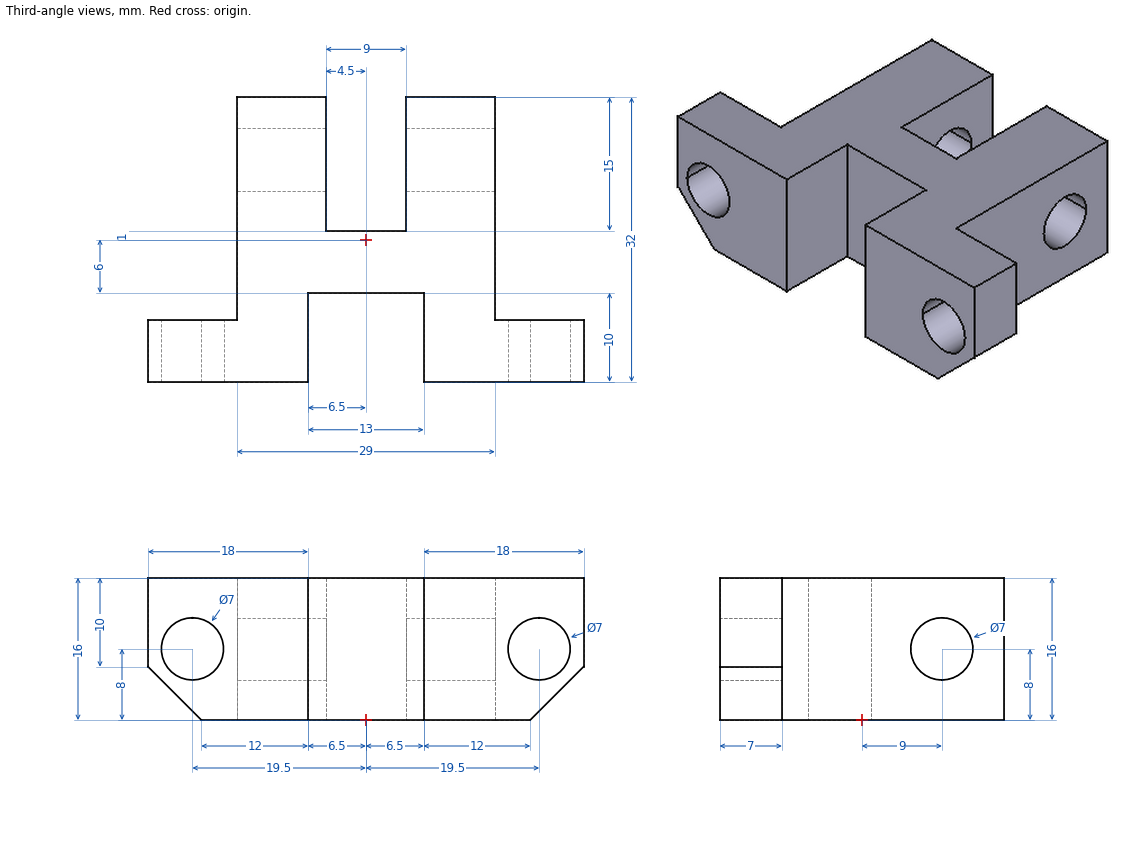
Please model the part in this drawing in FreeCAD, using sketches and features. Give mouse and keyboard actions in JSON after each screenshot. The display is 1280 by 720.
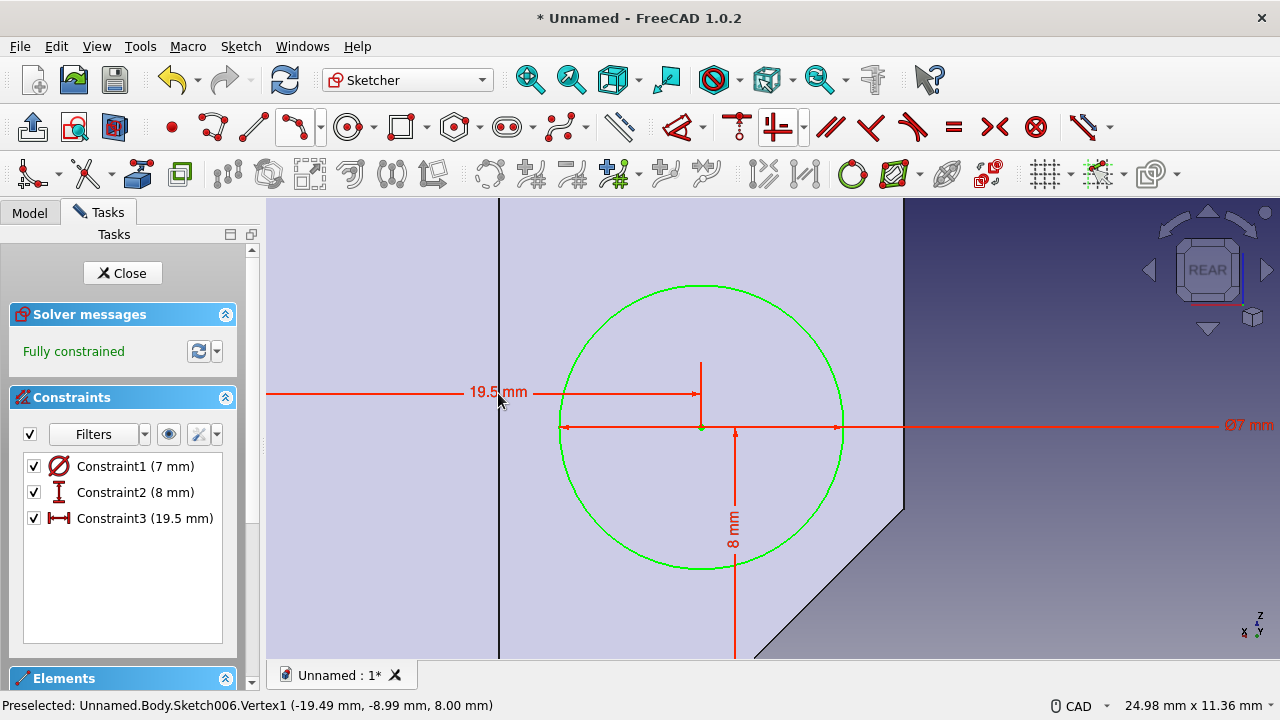
{"action": "left_click", "coordinate": [123, 273]}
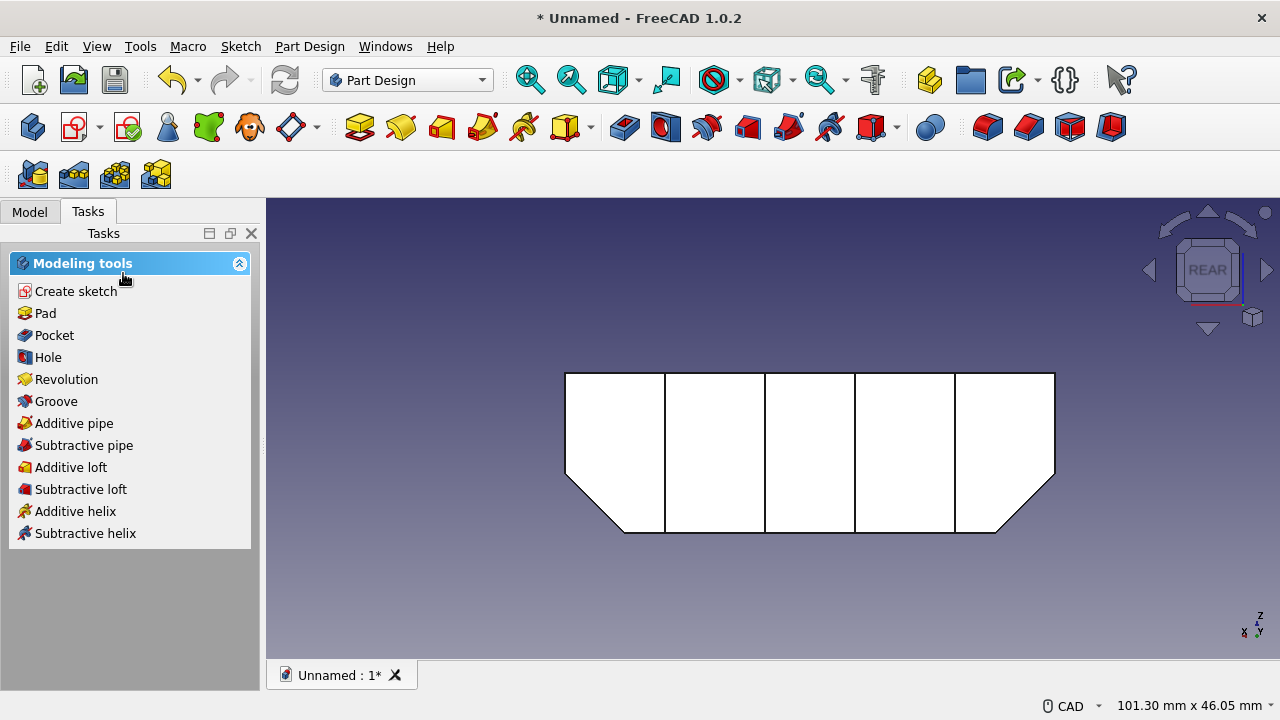
{"action": "left_click", "coordinate": [625, 128]}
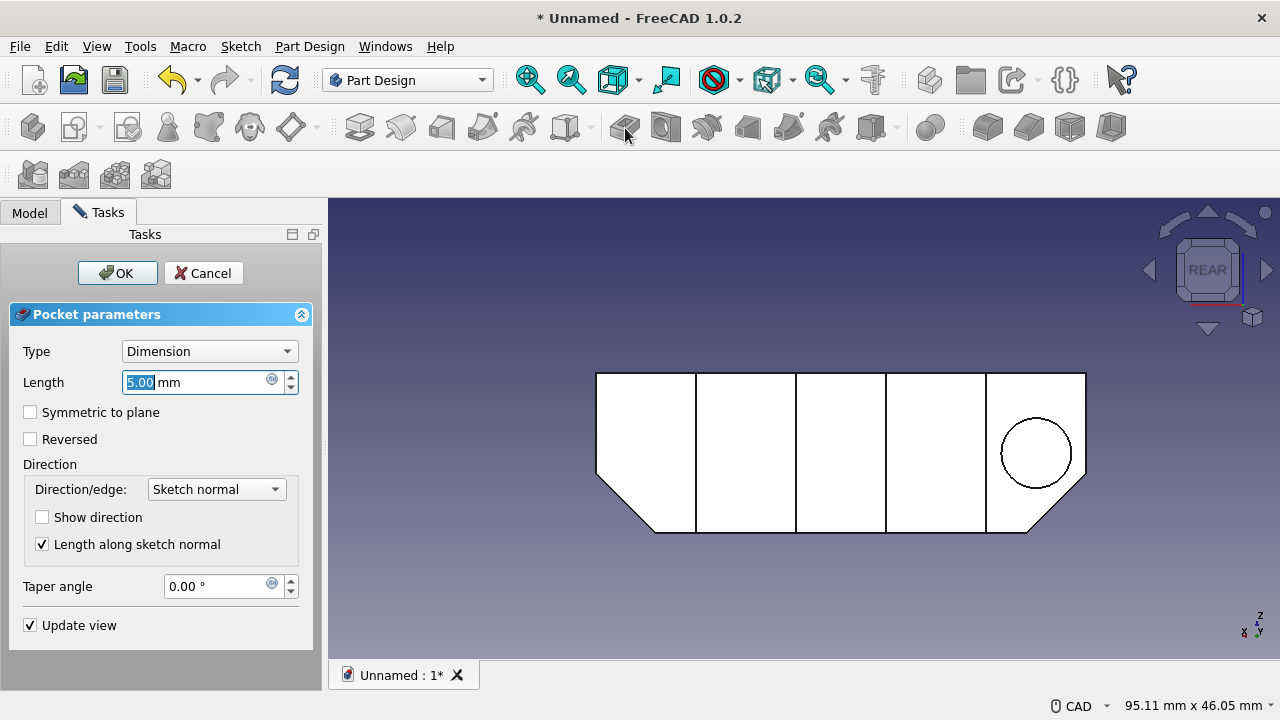
{"action": "type", "text": "7"}
{"action": "key", "text": "Tab"}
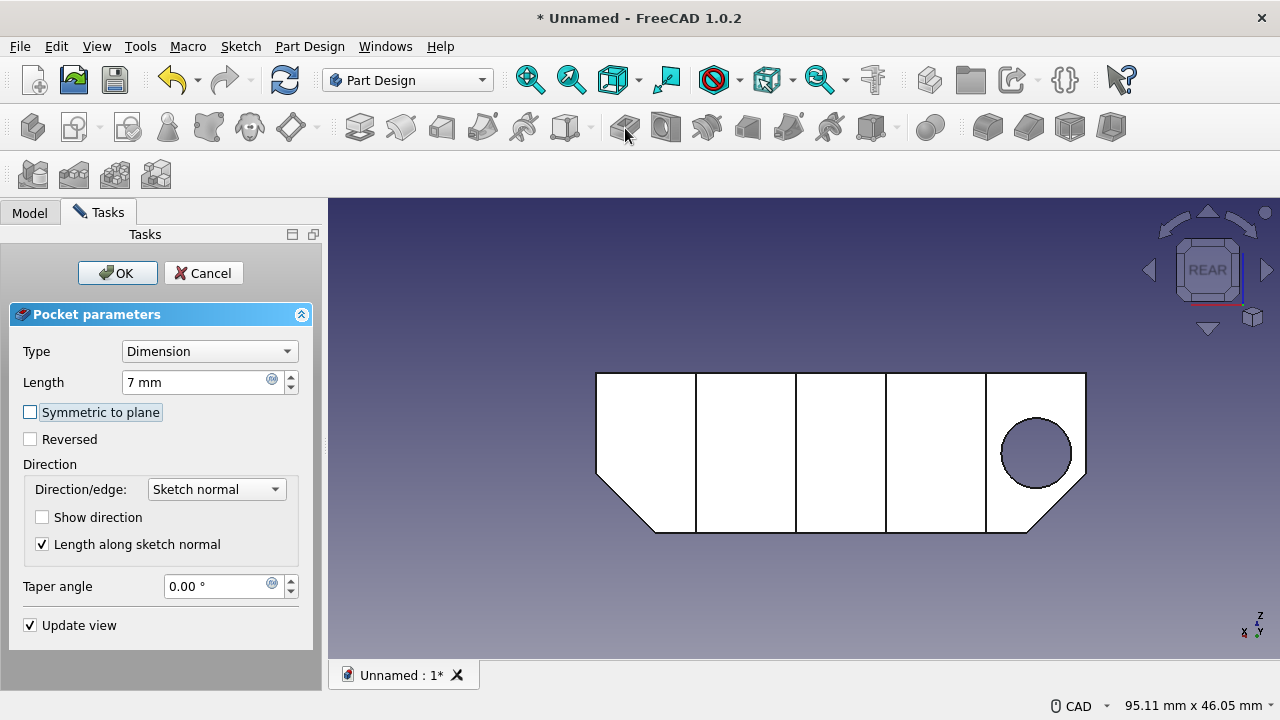
{"action": "left_click", "coordinate": [118, 273]}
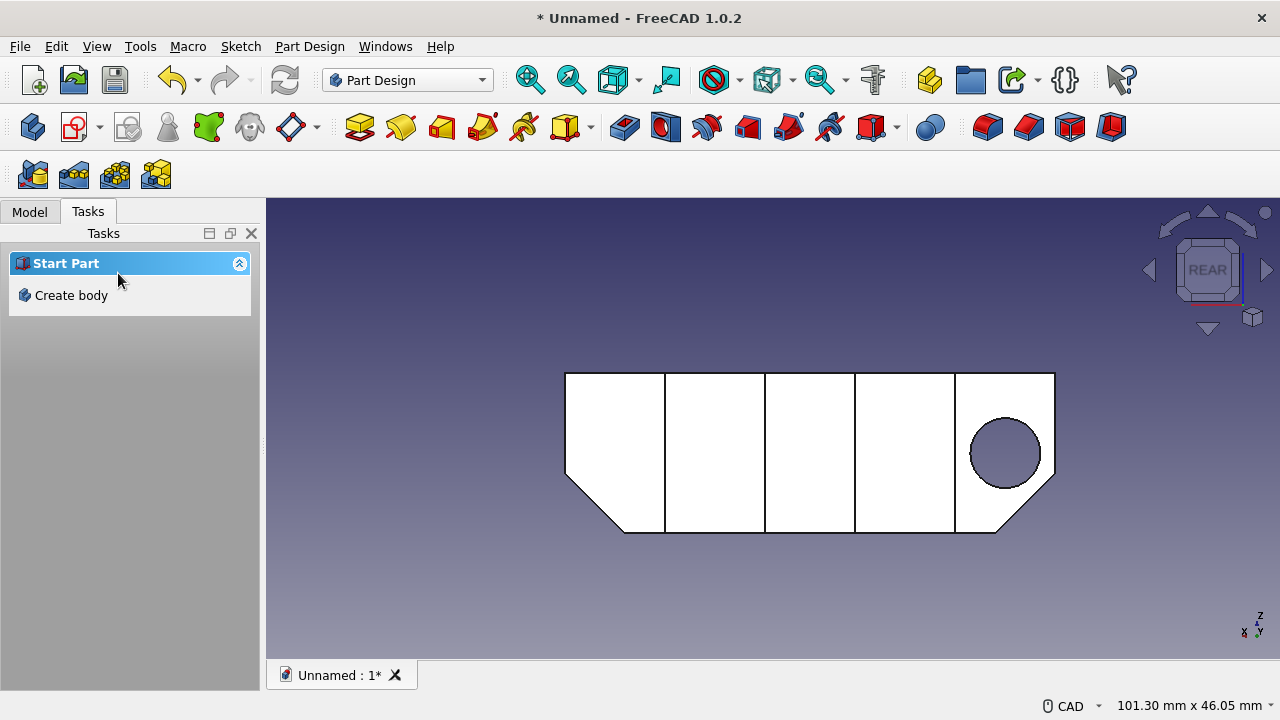
{"action": "left_click", "coordinate": [615, 429]}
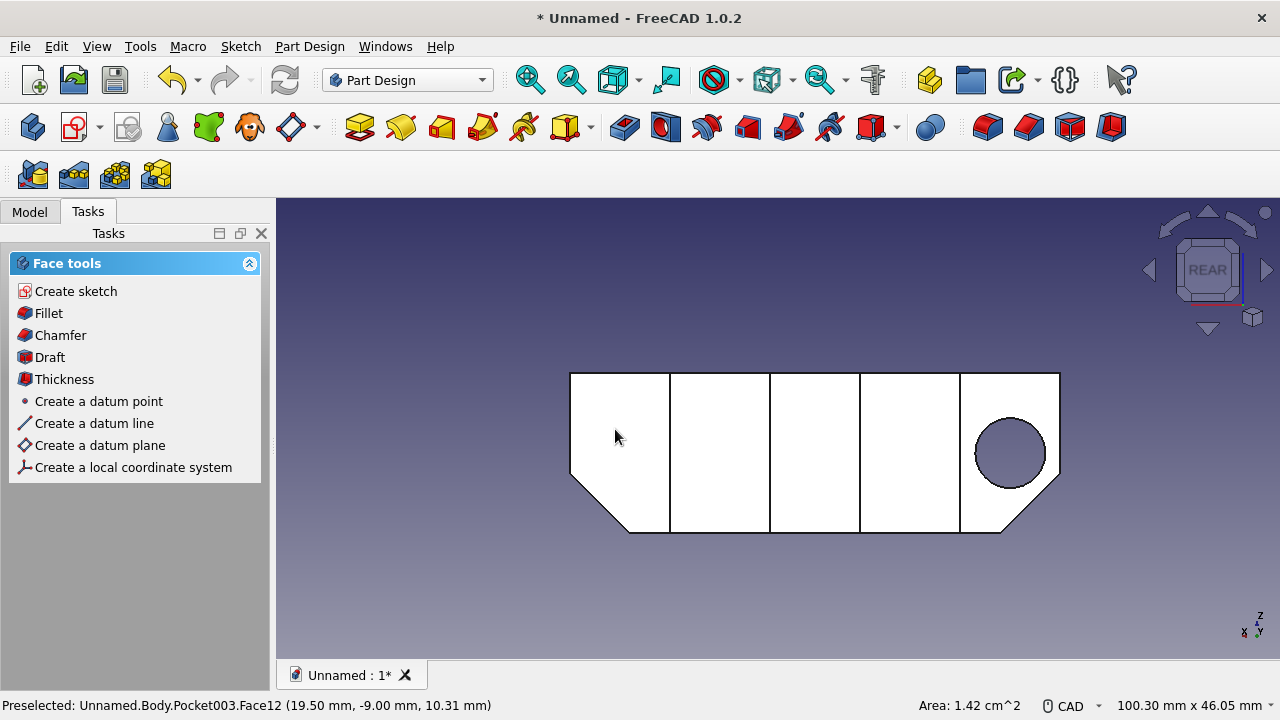
{"action": "left_click", "coordinate": [74, 128]}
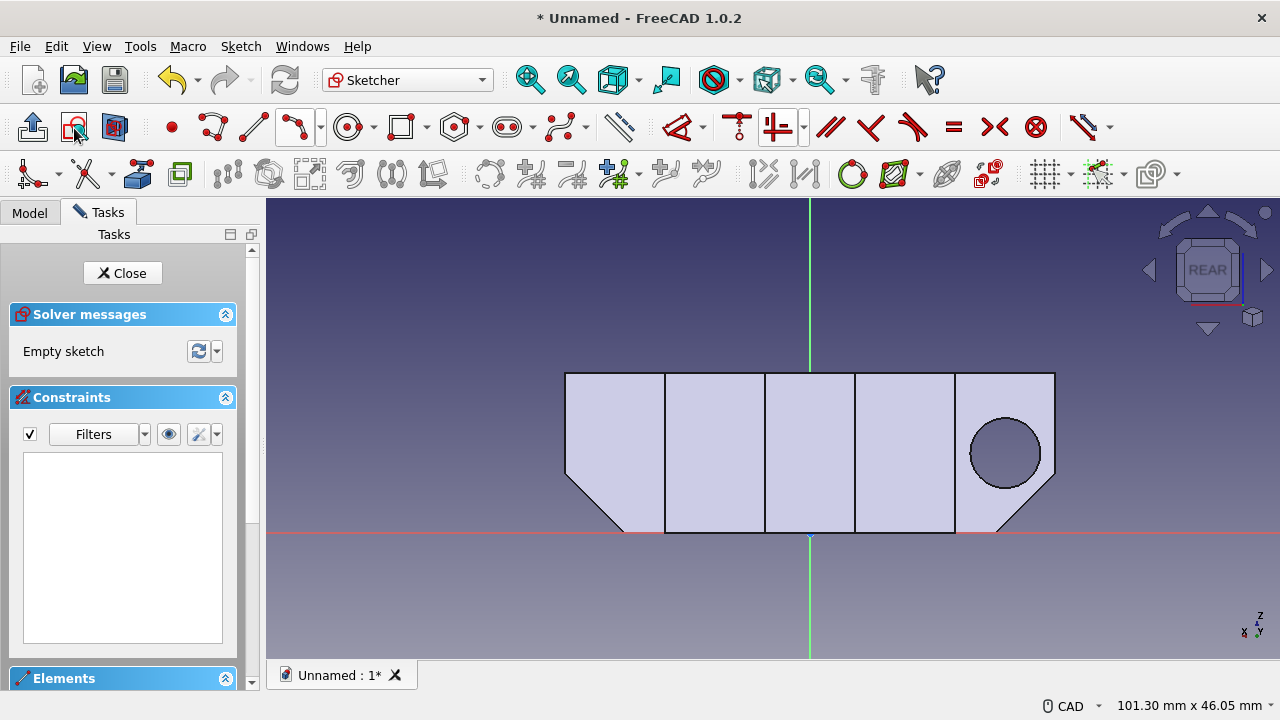
{"action": "scroll", "coordinate": [586, 461], "scroll_direction": "up", "scroll_amount": 7}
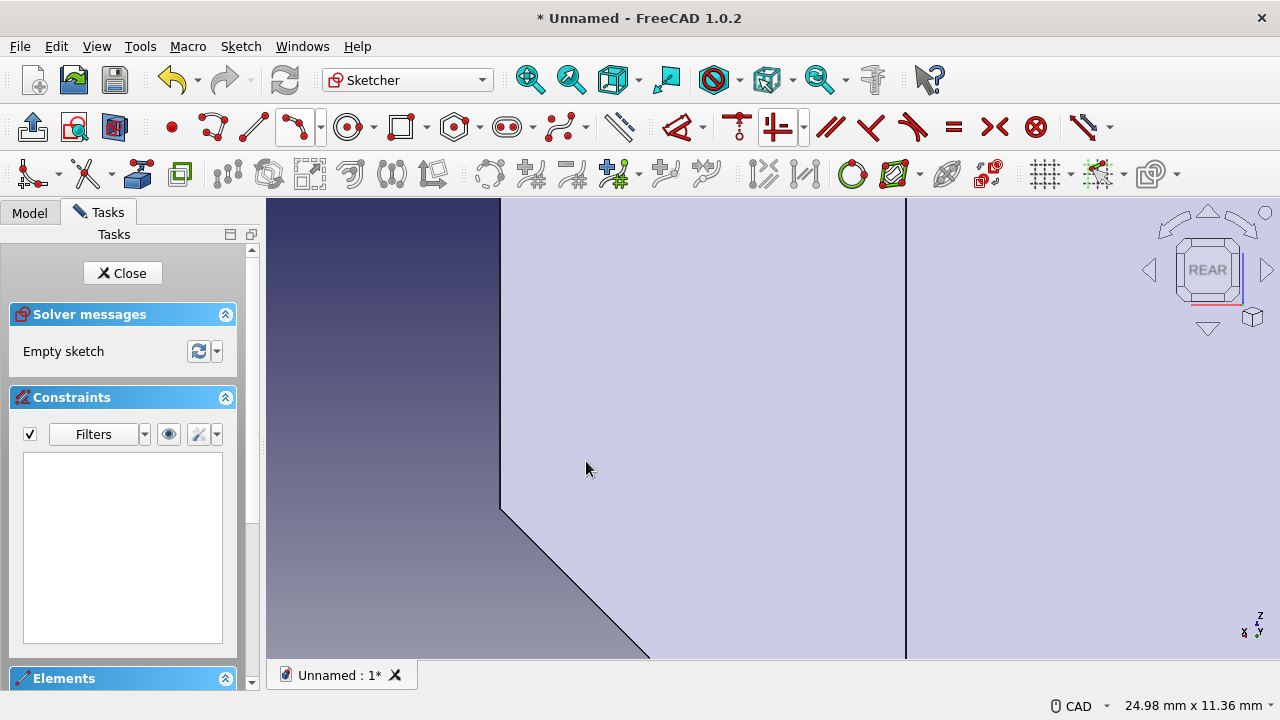
{"action": "left_click", "coordinate": [348, 128]}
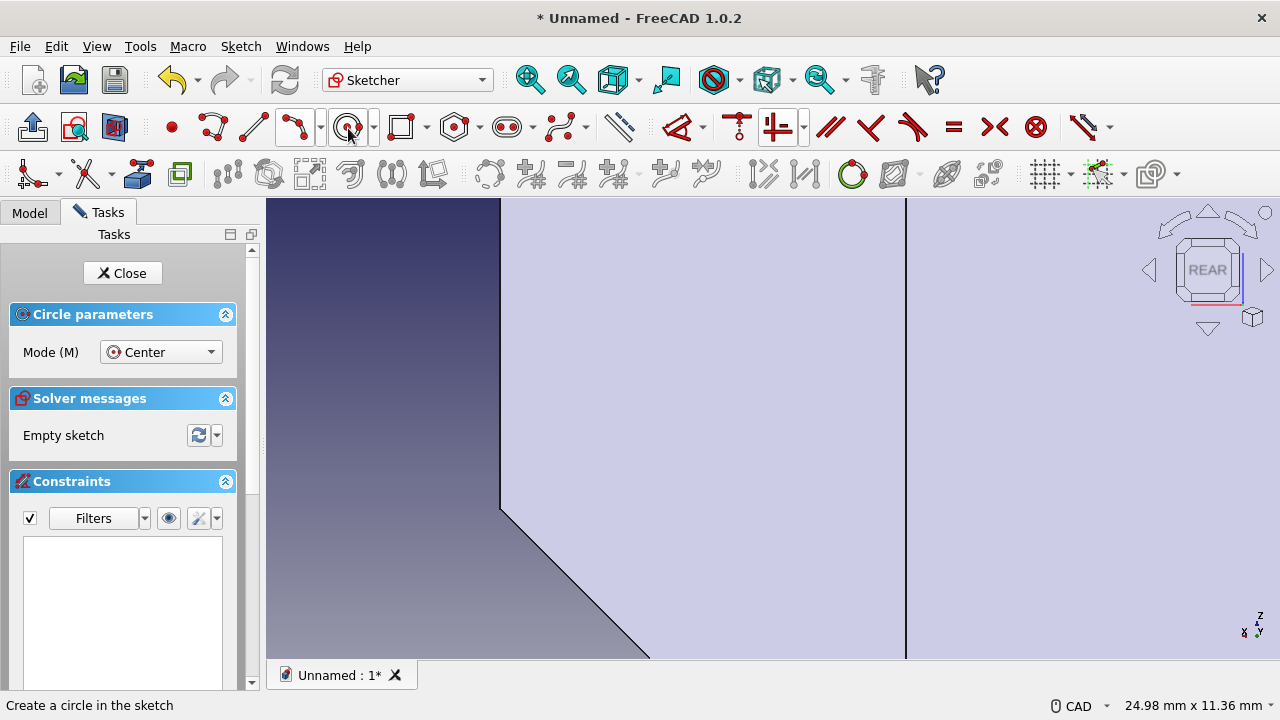
{"action": "left_click", "coordinate": [703, 427]}
{"action": "mouse_move", "coordinate": [803, 327]}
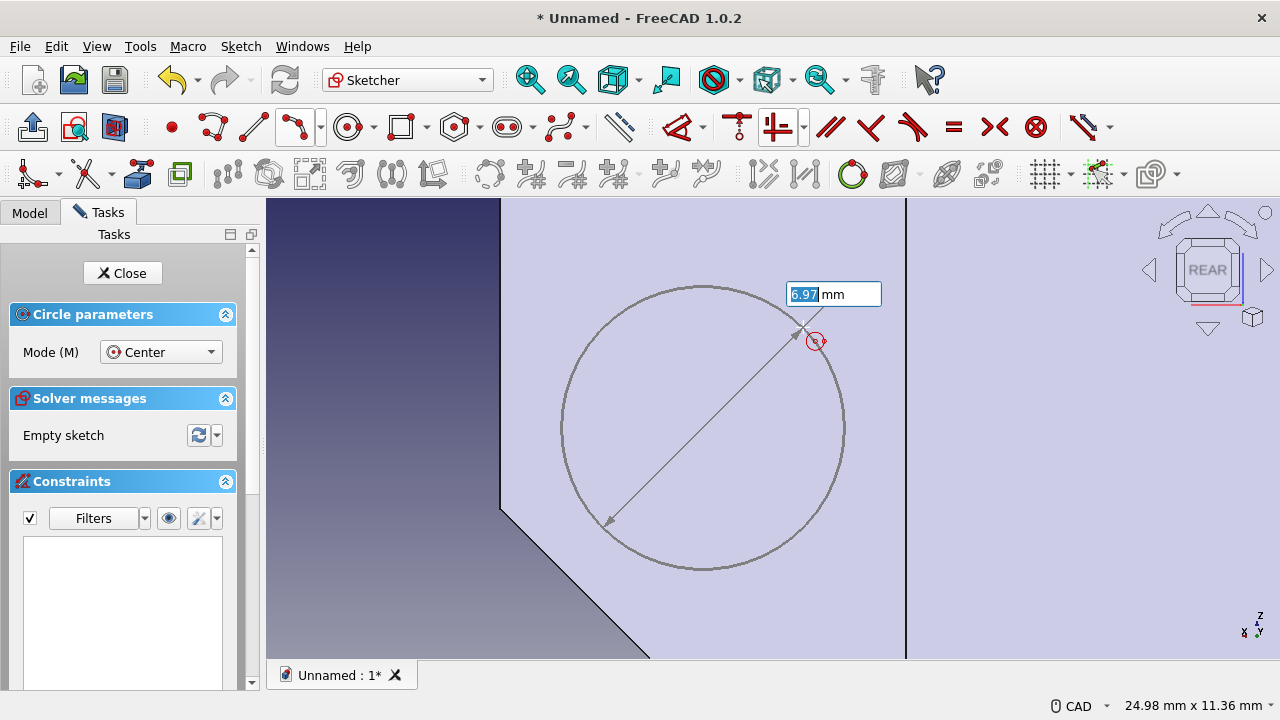
{"action": "type", "text": "7"}
{"action": "key", "text": "Return"}
{"action": "key", "text": "Escape"}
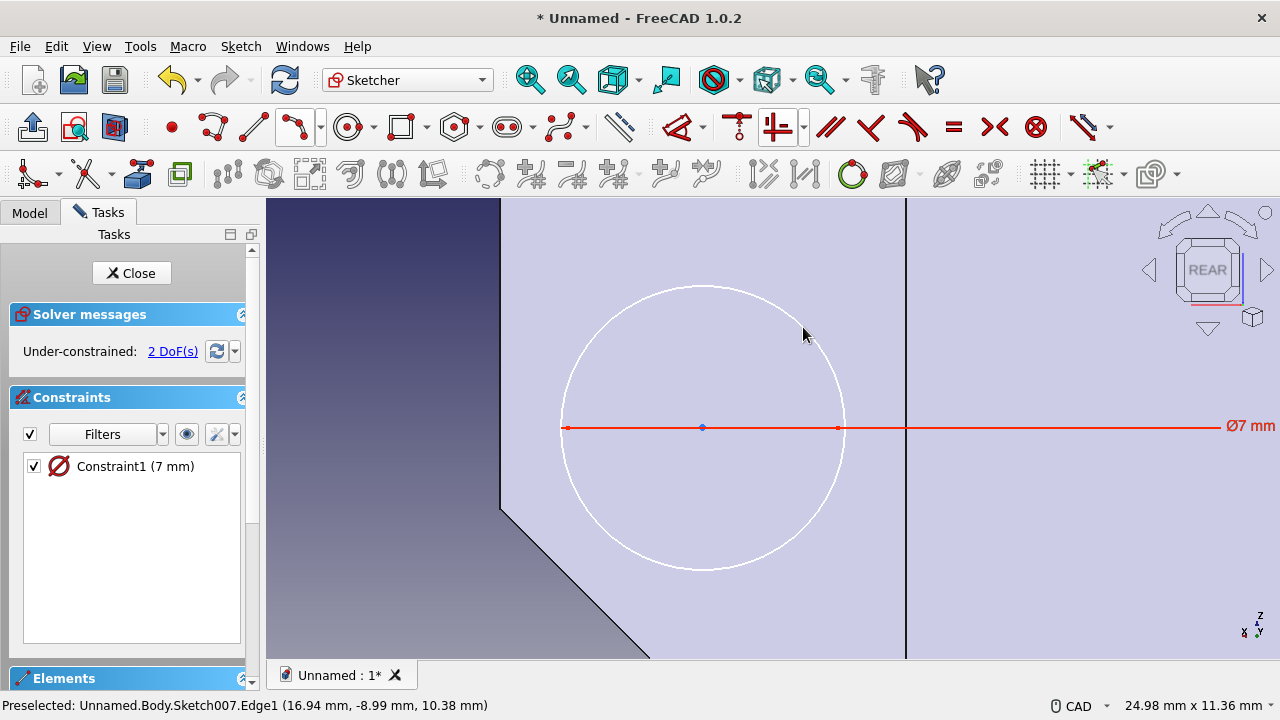
{"action": "left_click", "coordinate": [676, 128]}